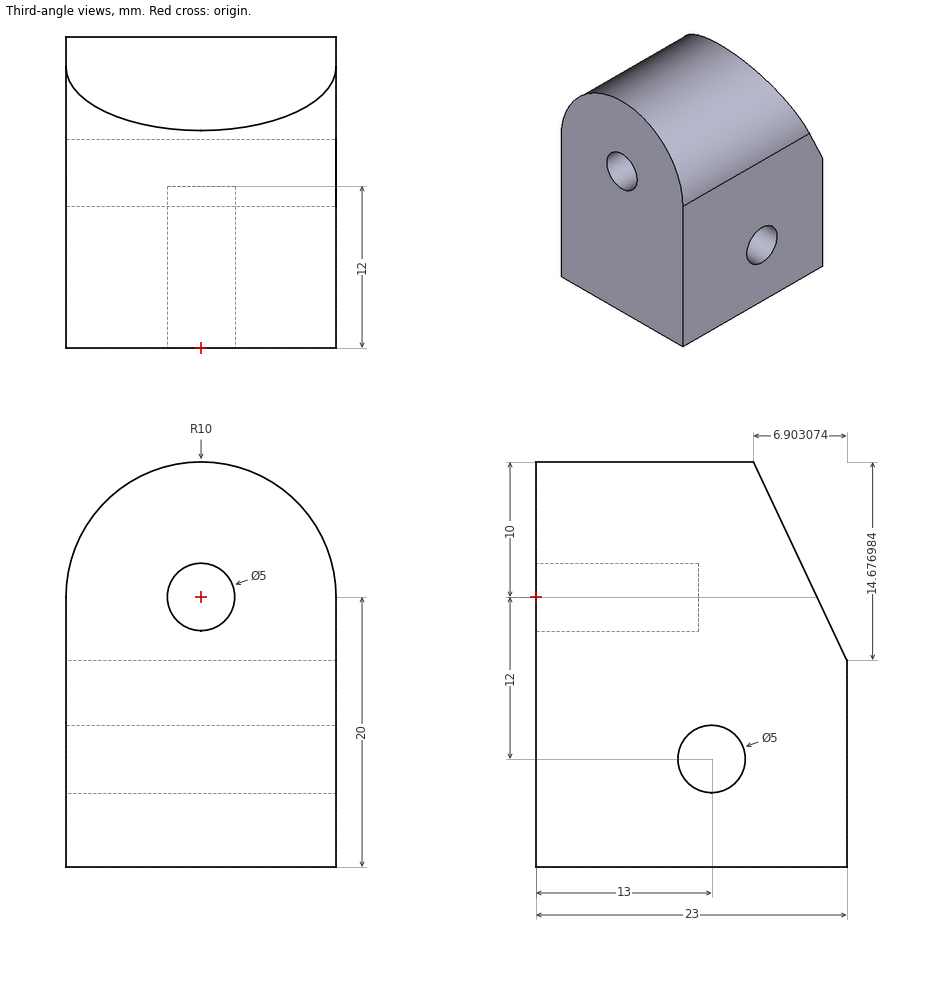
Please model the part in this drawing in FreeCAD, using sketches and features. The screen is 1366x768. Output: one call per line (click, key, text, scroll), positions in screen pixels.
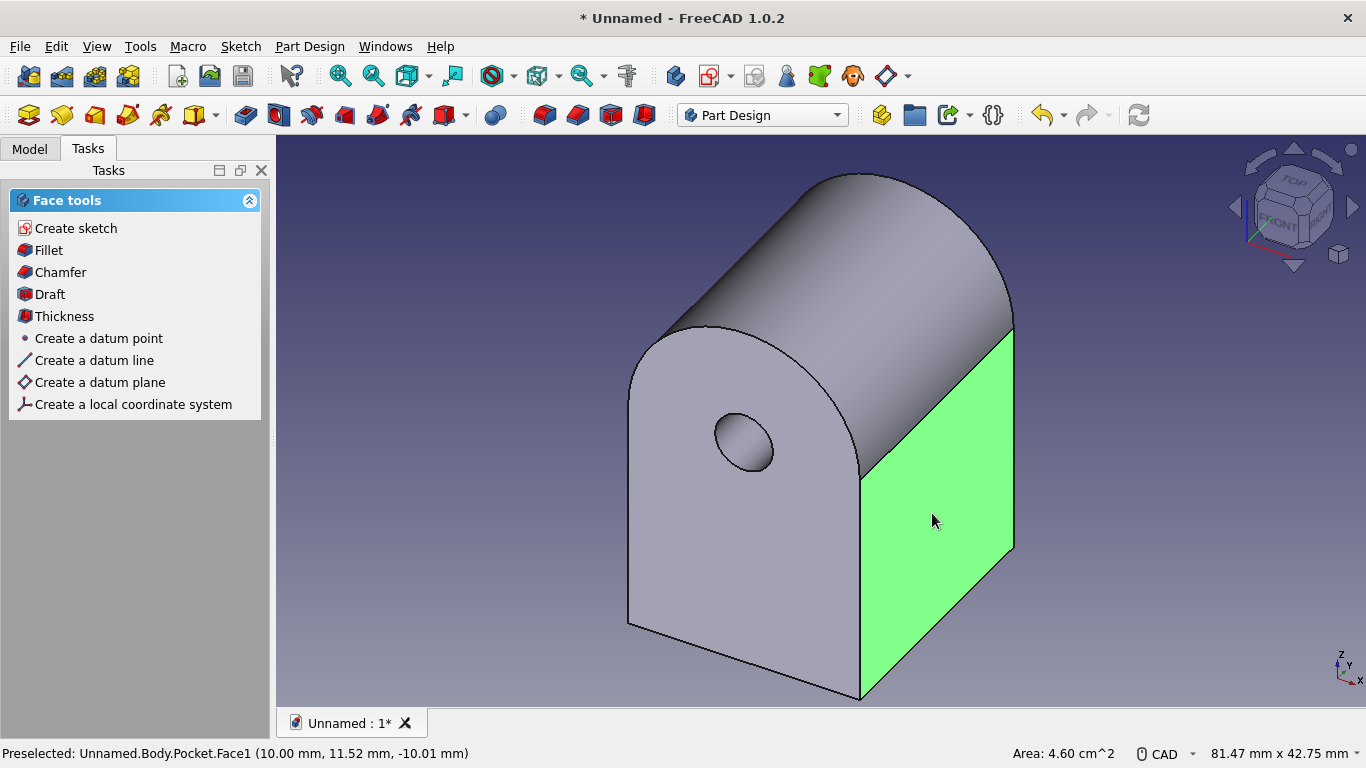
click(708, 76)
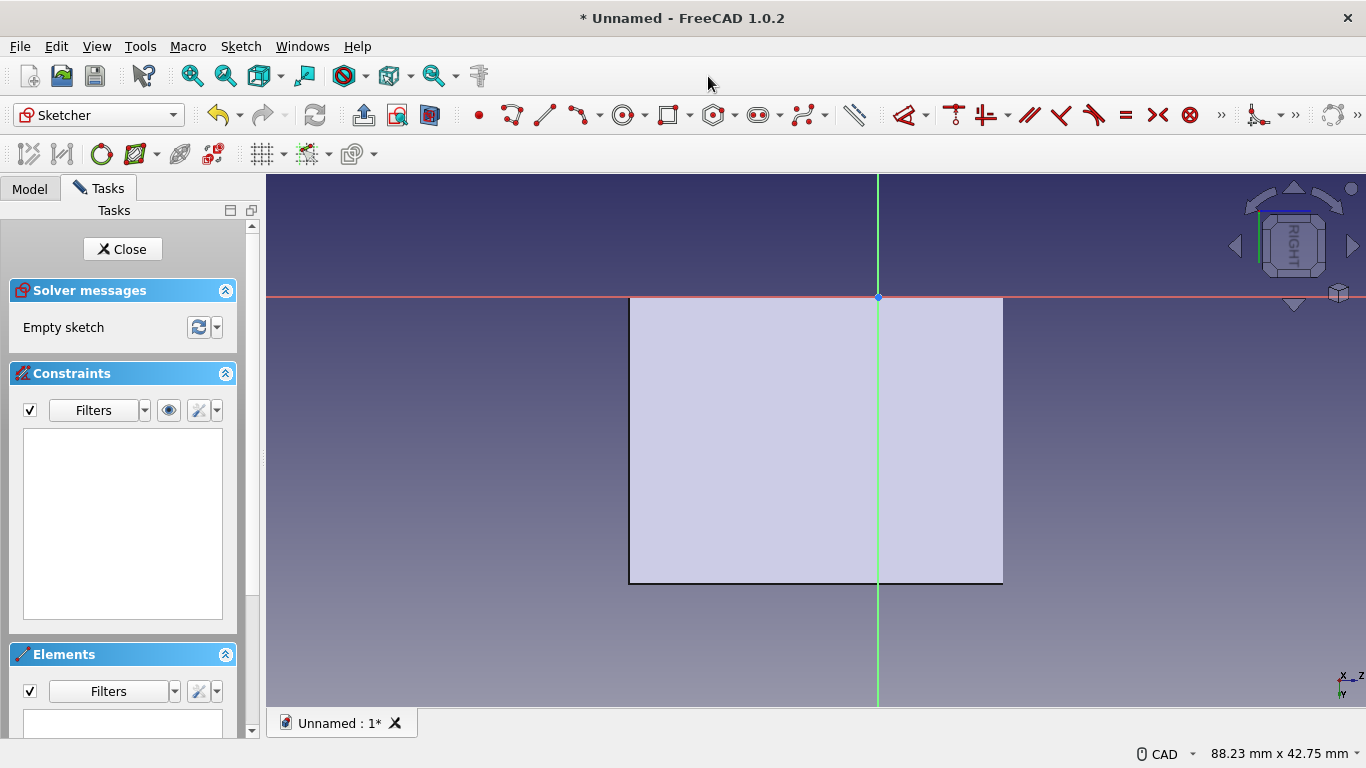
scroll(724, 464, up, 8)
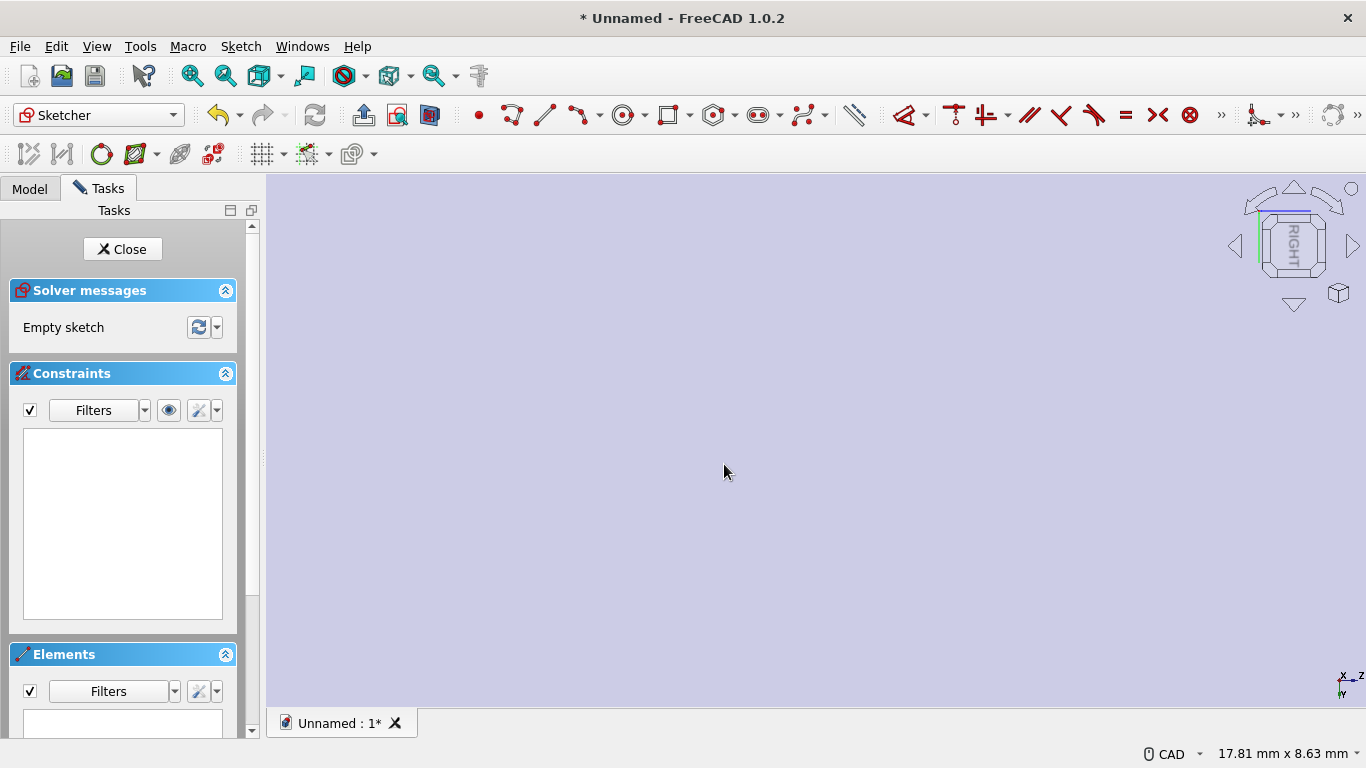
key(g)
key(c)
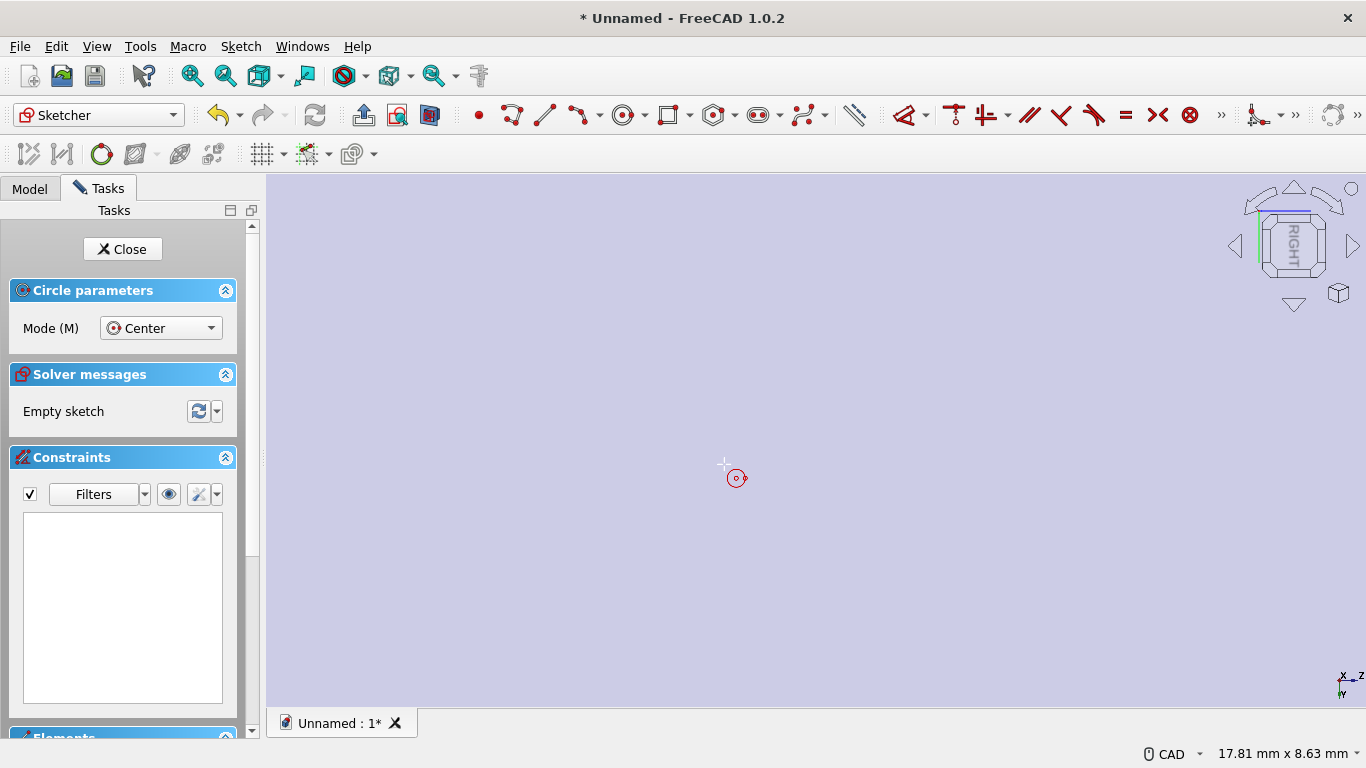
click(746, 438)
click(856, 329)
key(Escape)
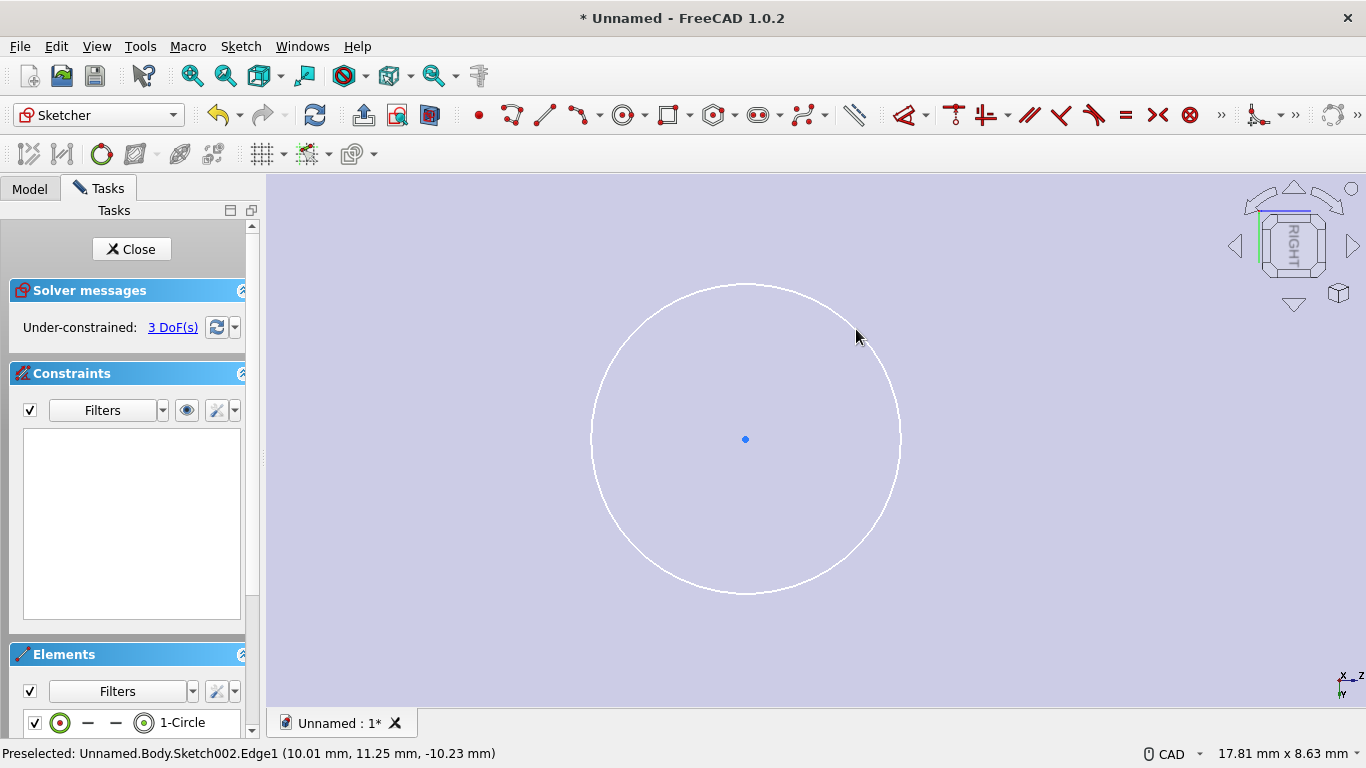
click(904, 116)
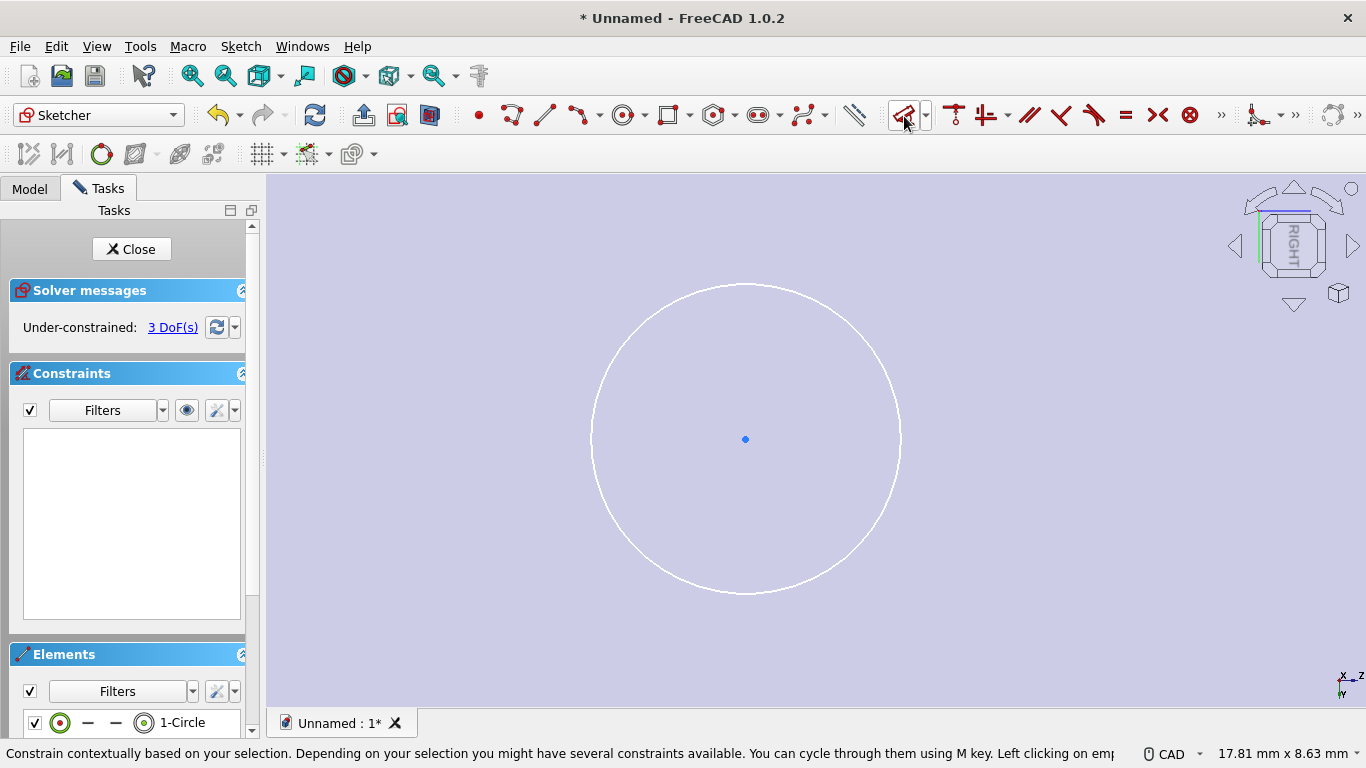
click(855, 329)
click(878, 306)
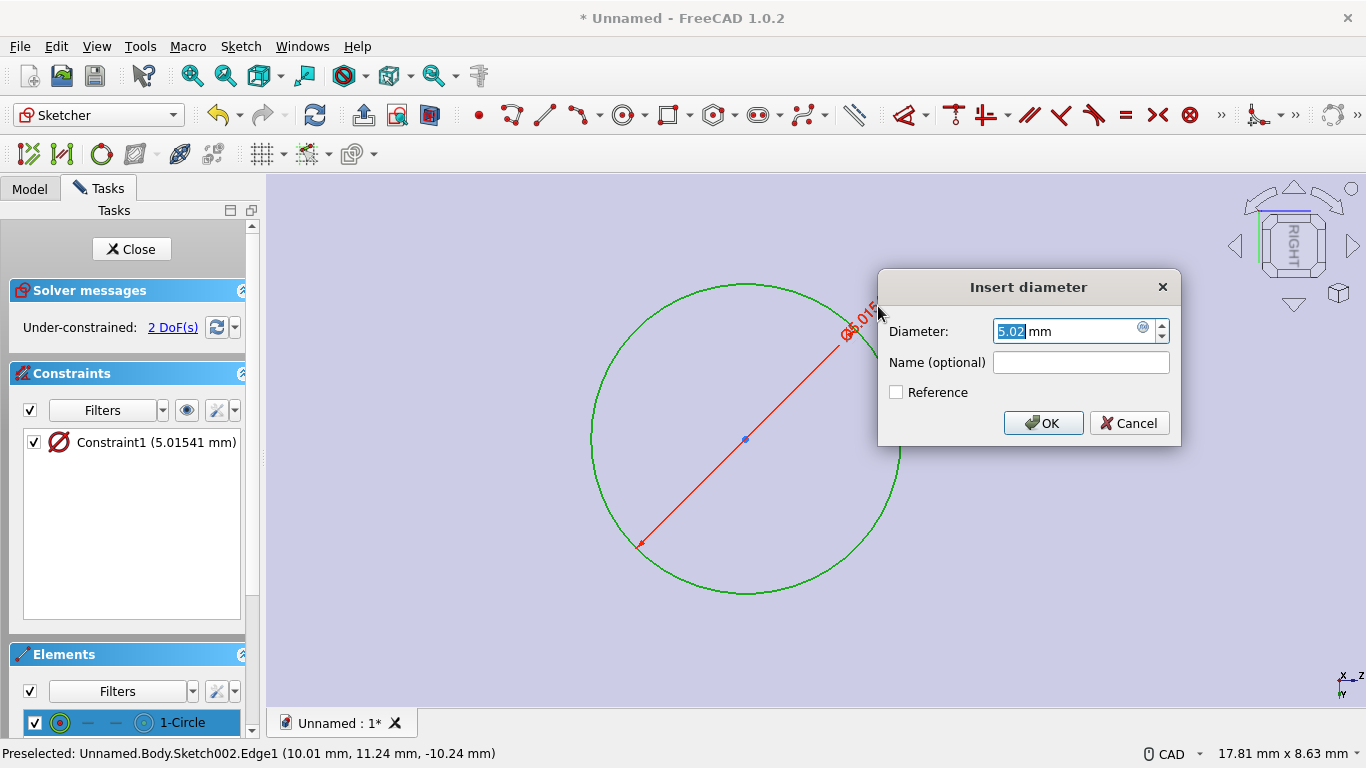
text(5)
key(Return)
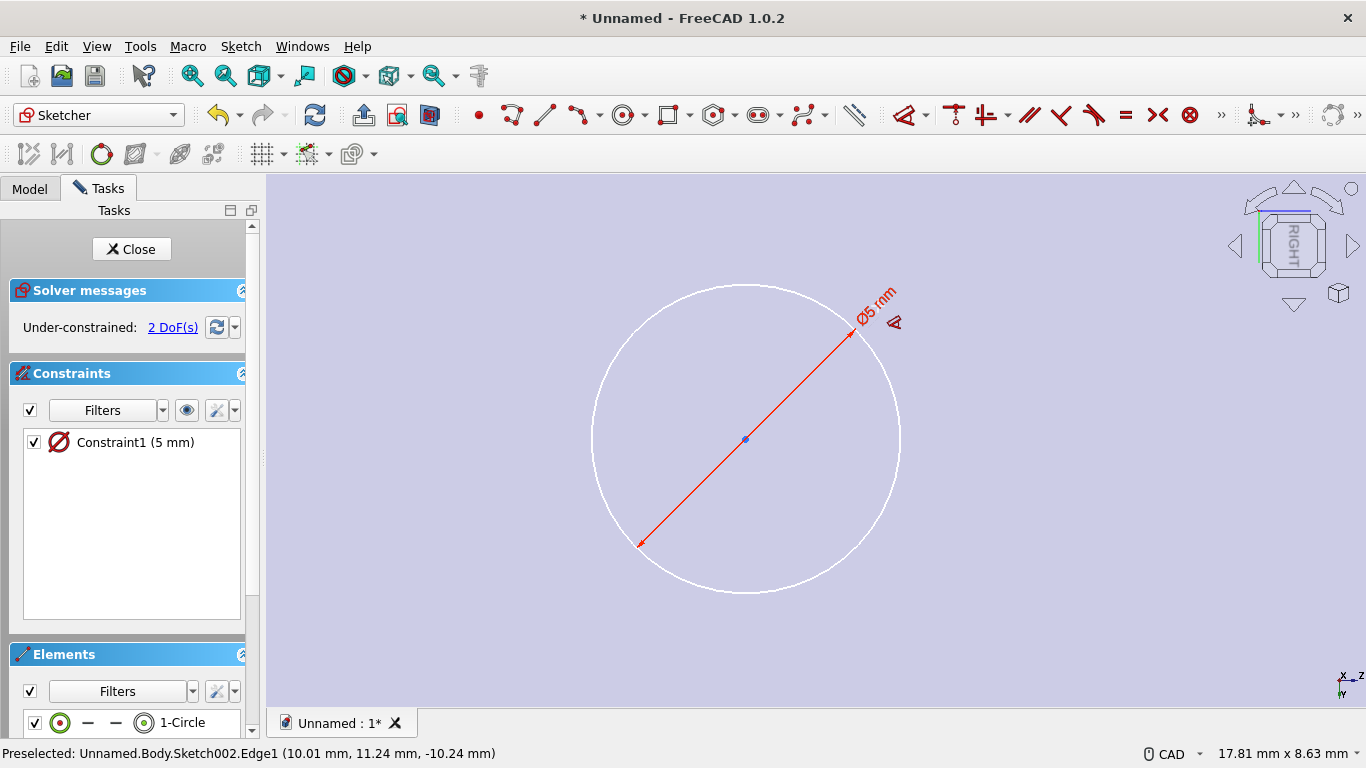
click(746, 439)
click(974, 473)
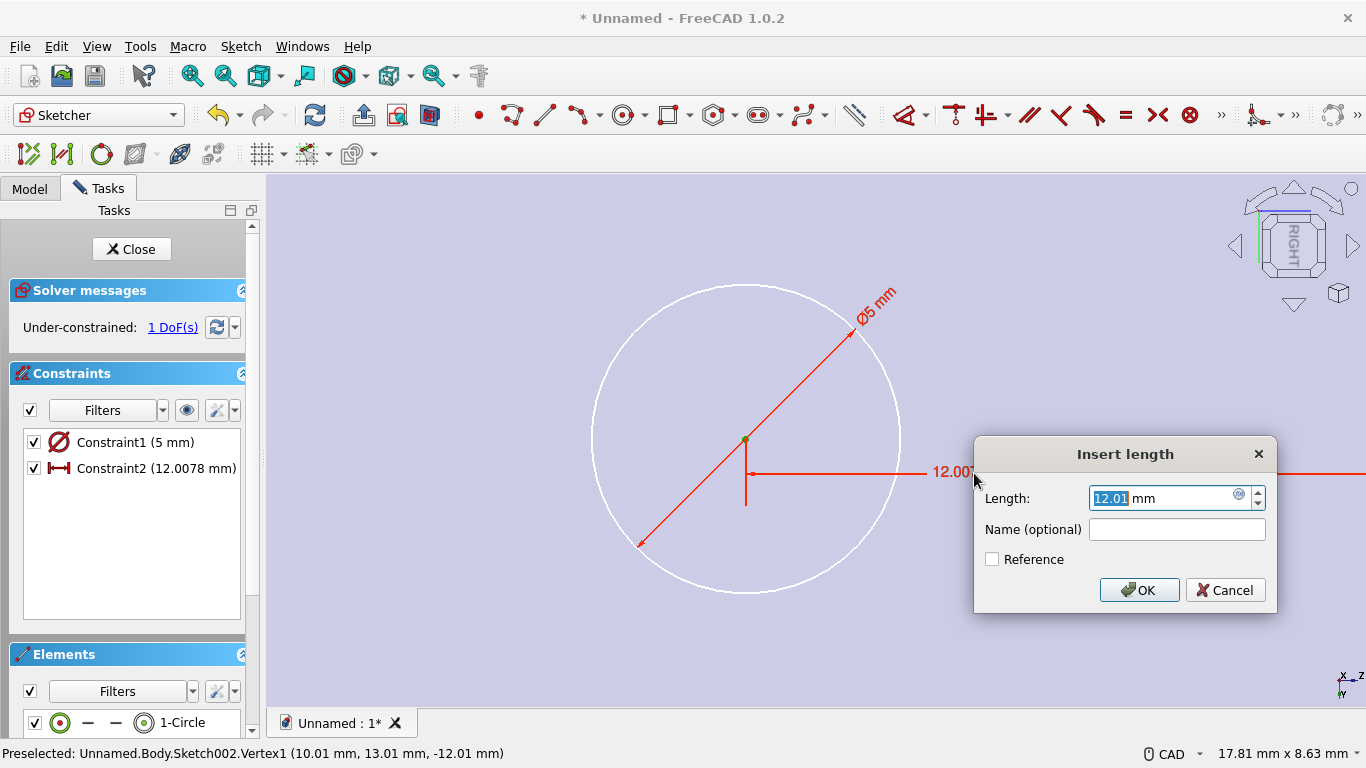
text(12)
key(Return)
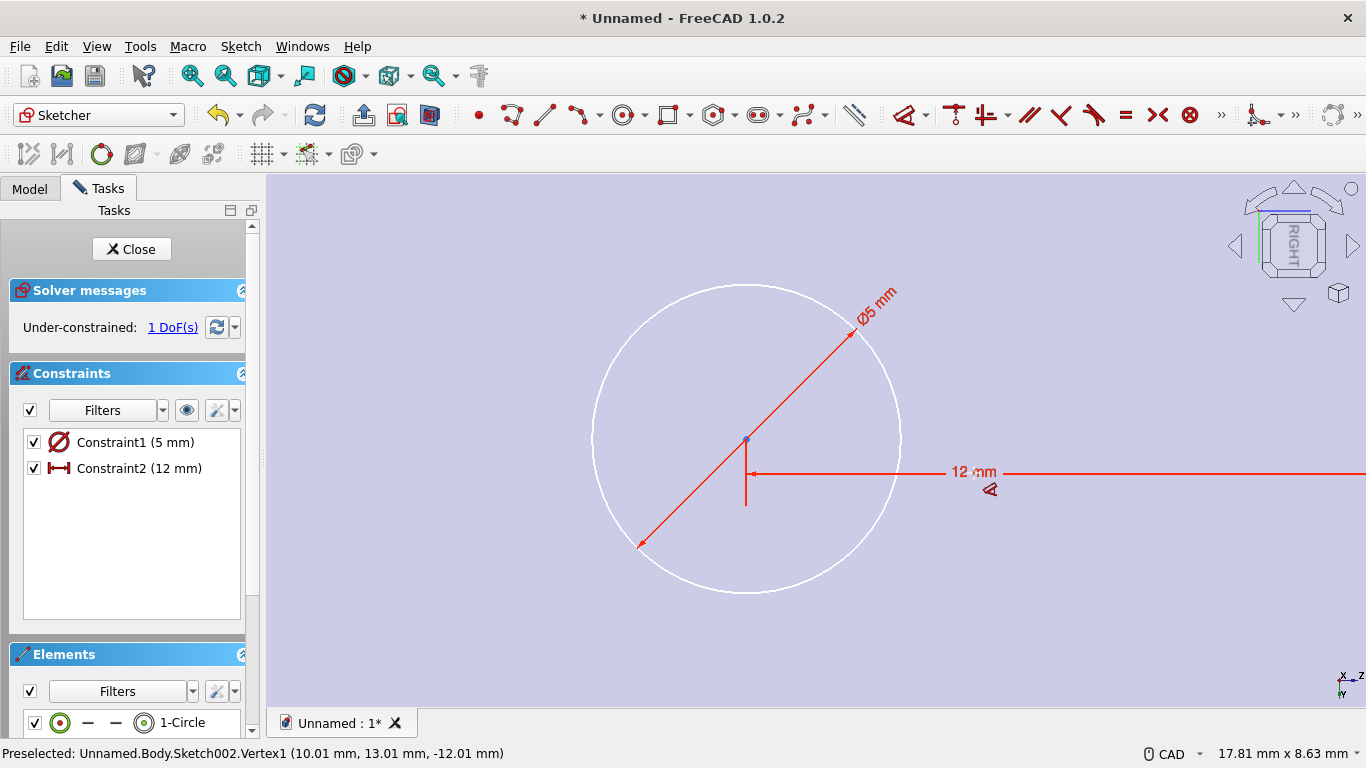
click(746, 439)
click(712, 321)